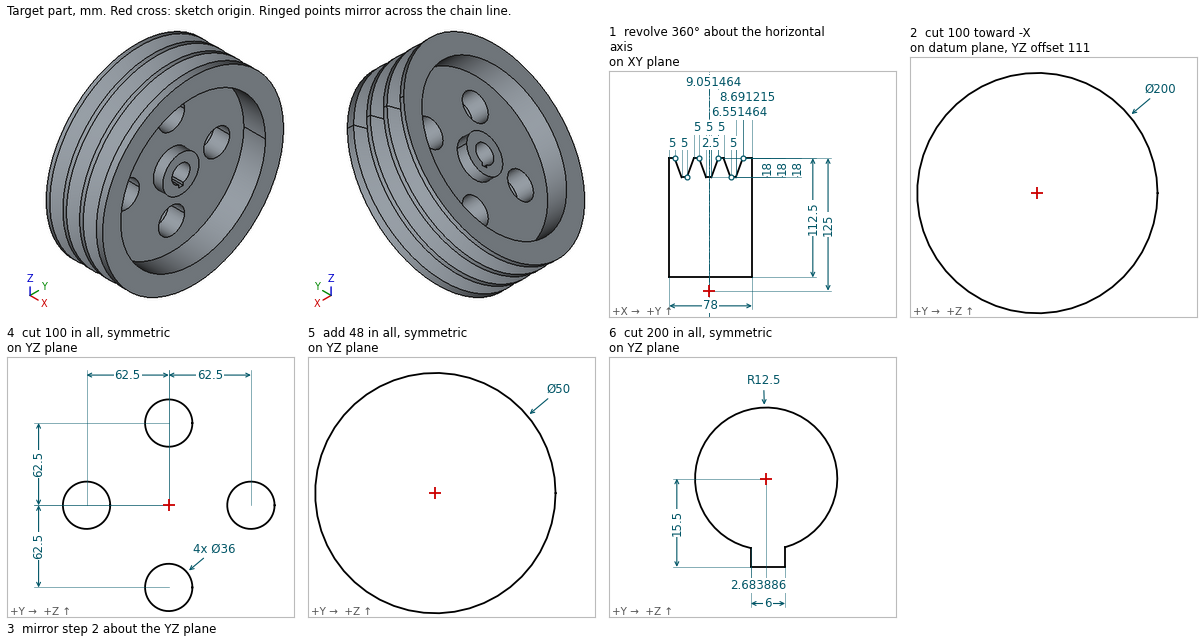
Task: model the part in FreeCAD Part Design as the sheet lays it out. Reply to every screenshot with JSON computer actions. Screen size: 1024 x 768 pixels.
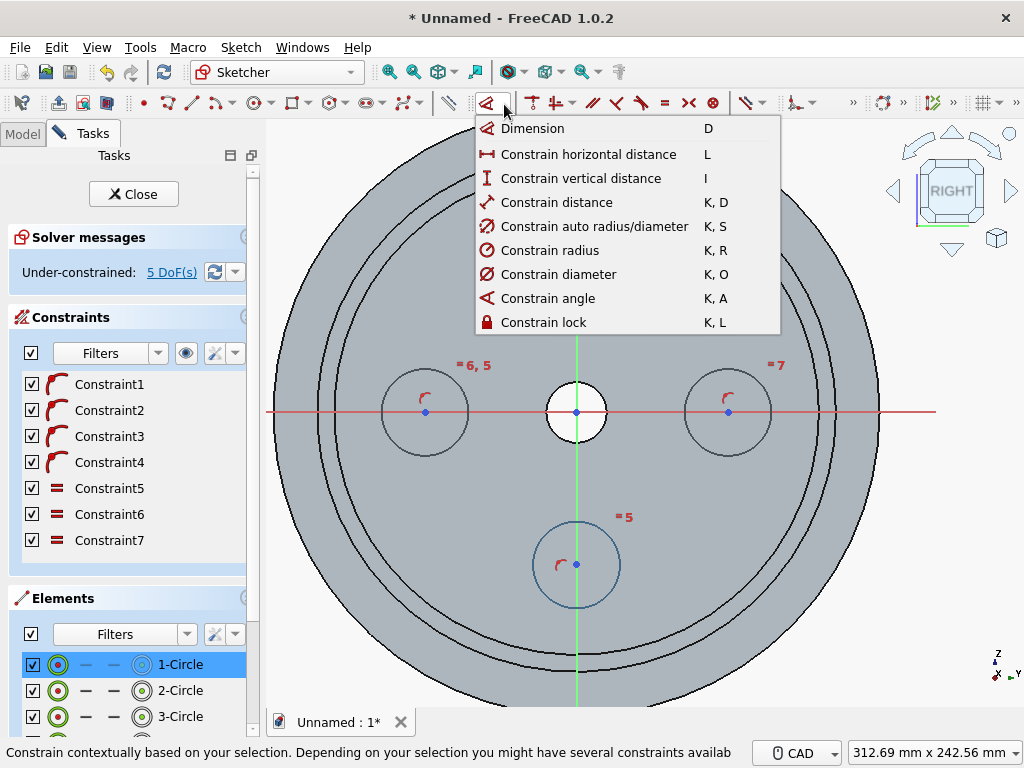
{"action": "left_click", "coordinate": [628, 274]}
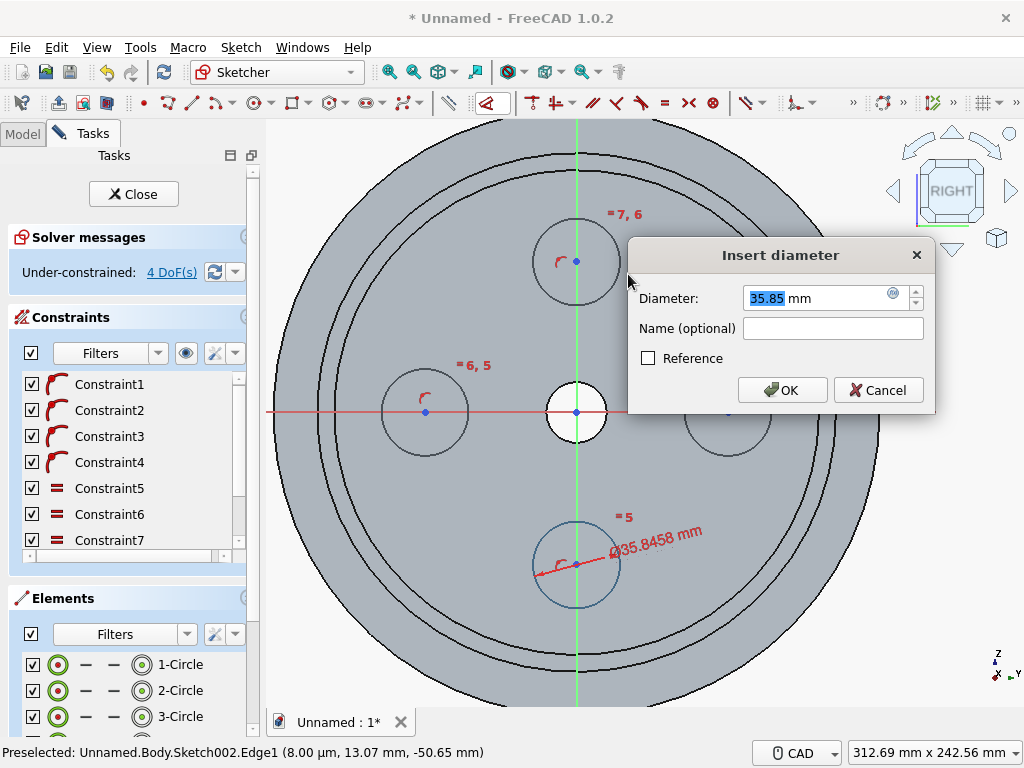
{"action": "type", "text": "36"}
{"action": "key", "text": "Return"}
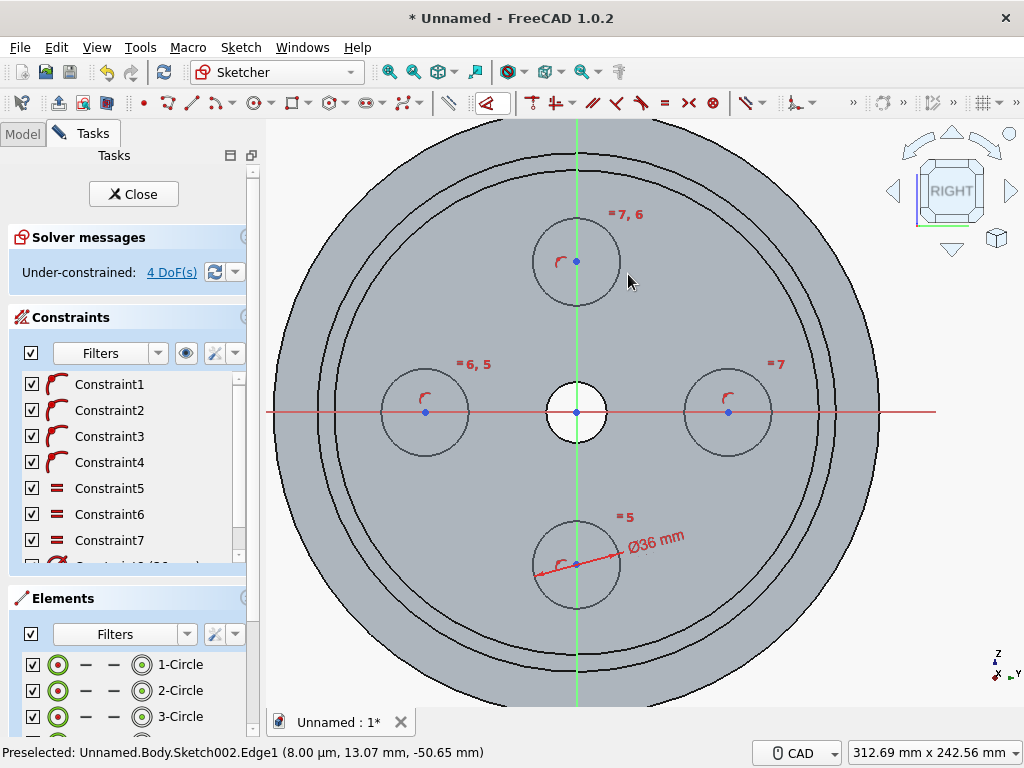
{"action": "left_click", "coordinate": [577, 565]}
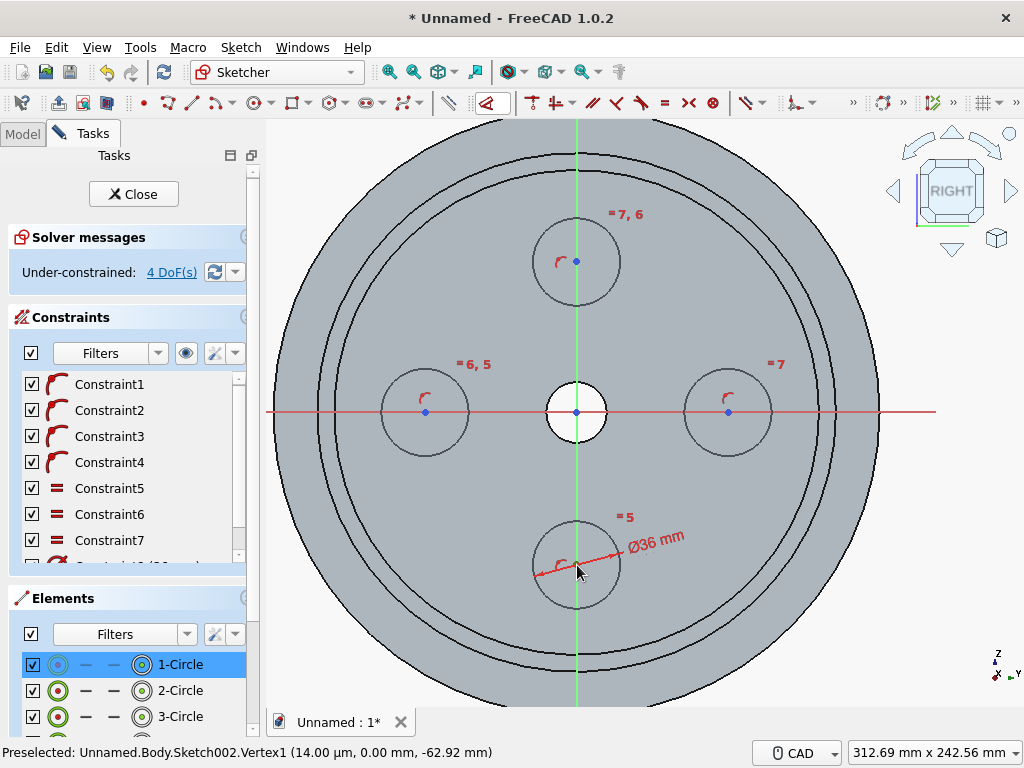
{"action": "key", "text": "i"}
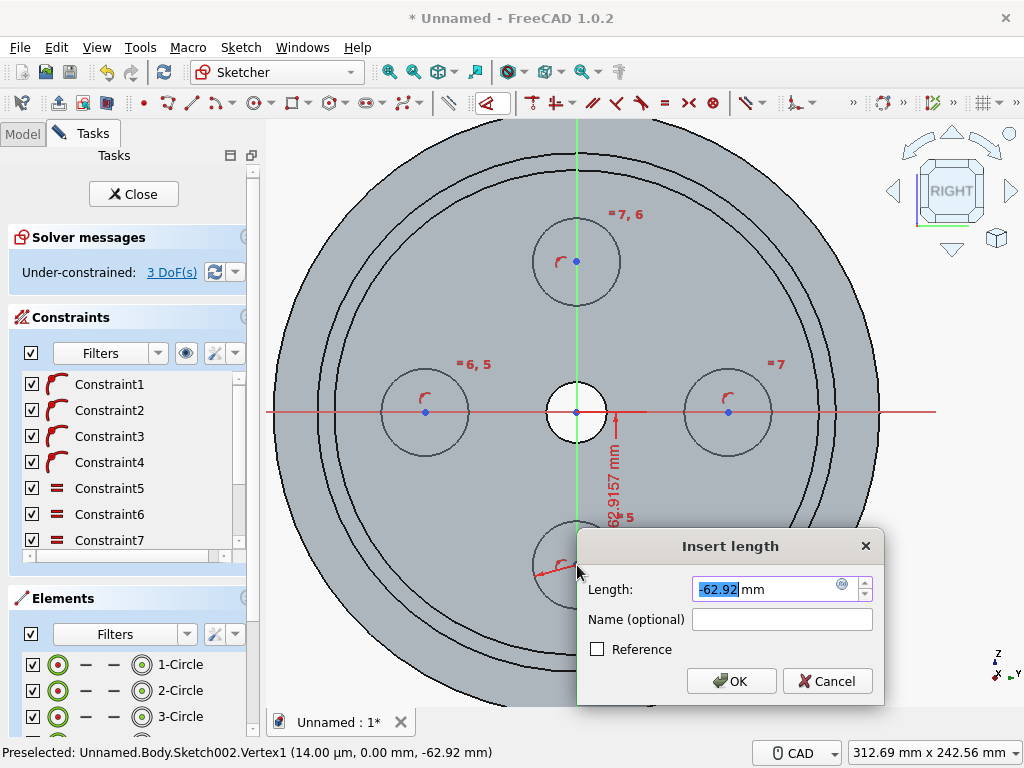
{"action": "type", "text": "-62.5"}
{"action": "key", "text": "Return"}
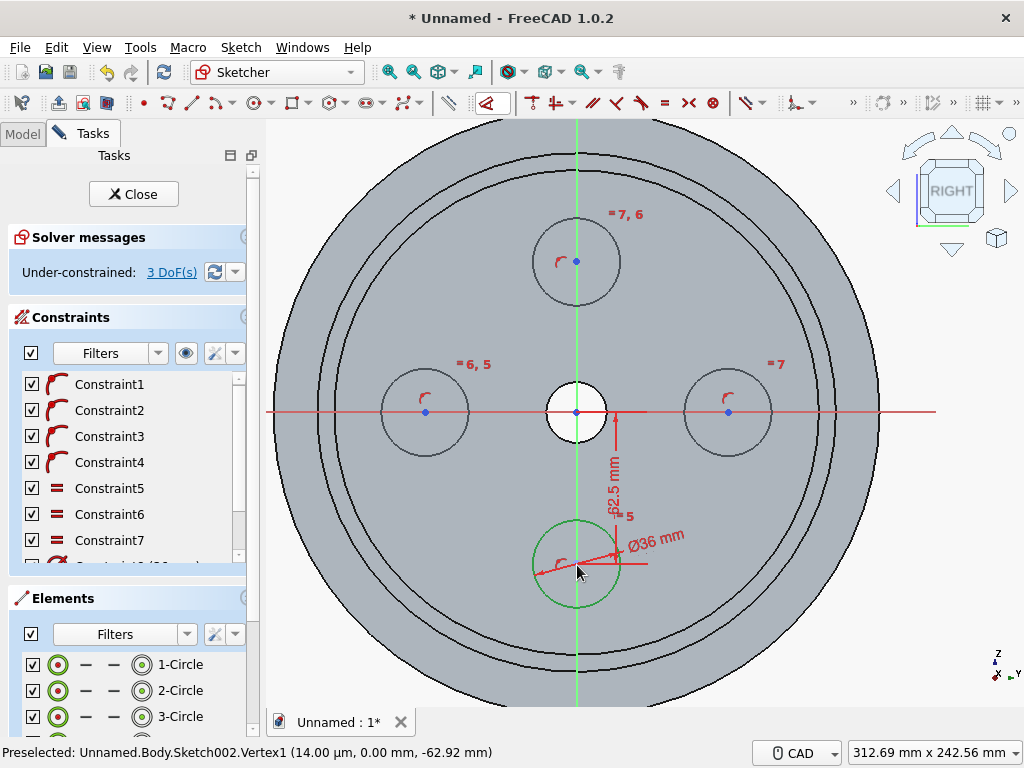
{"action": "left_click", "coordinate": [425, 412]}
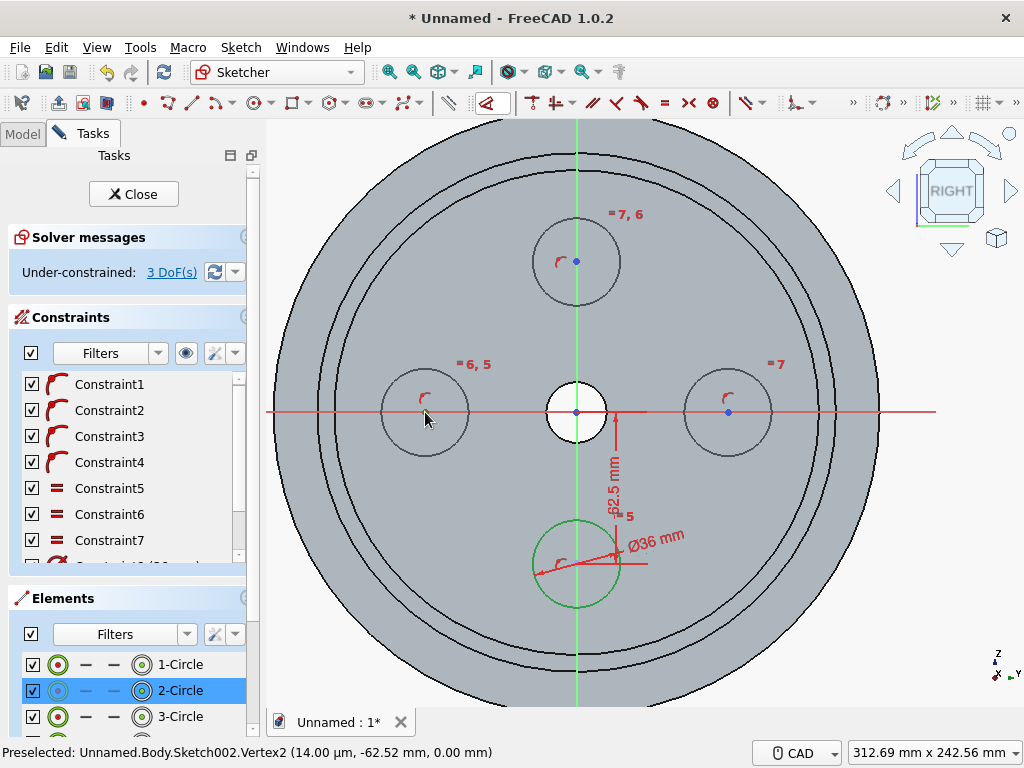
{"action": "left_click", "coordinate": [504, 104]}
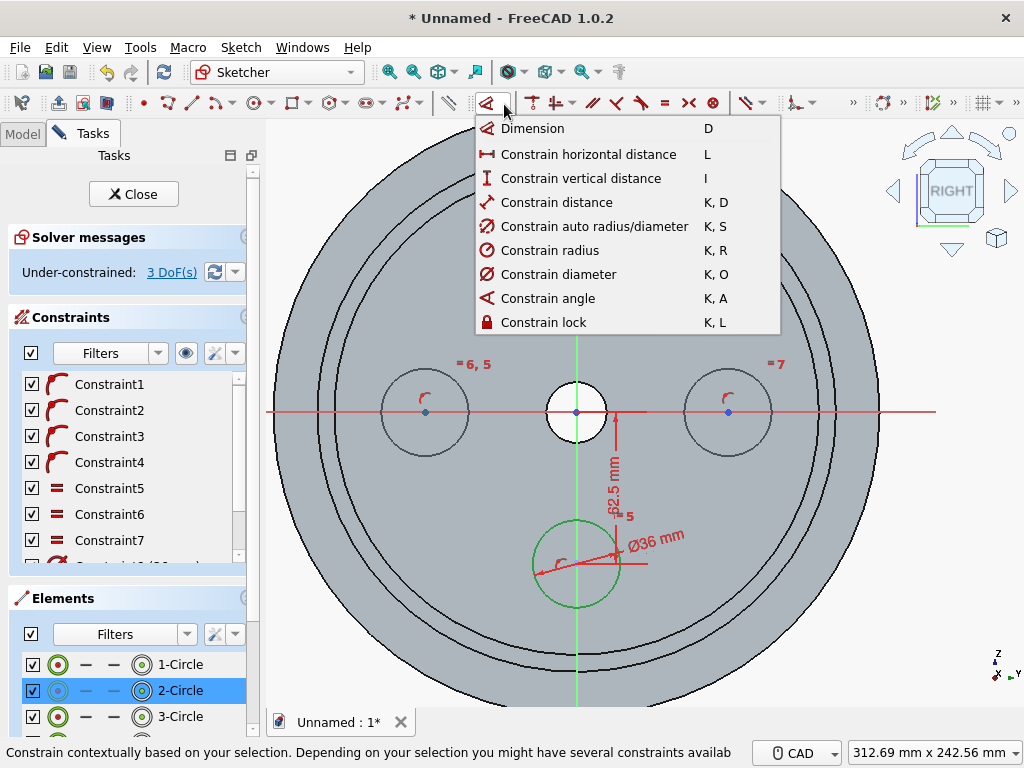
{"action": "left_click", "coordinate": [628, 154]}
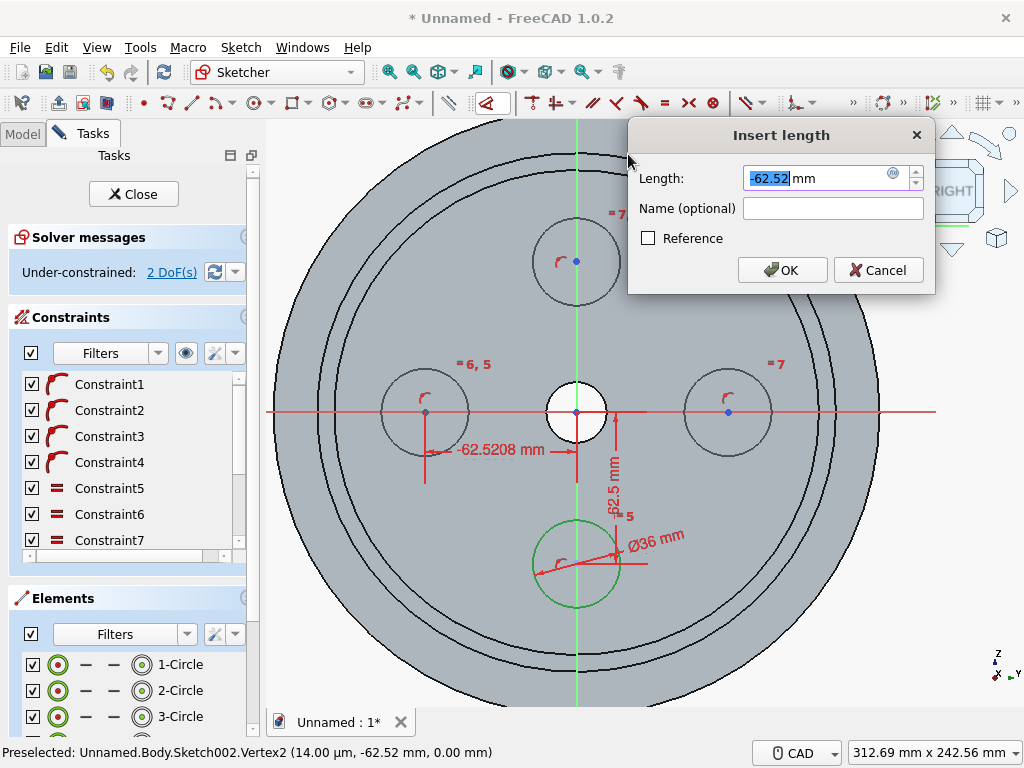
{"action": "type", "text": "-62.5"}
{"action": "key", "text": "Return"}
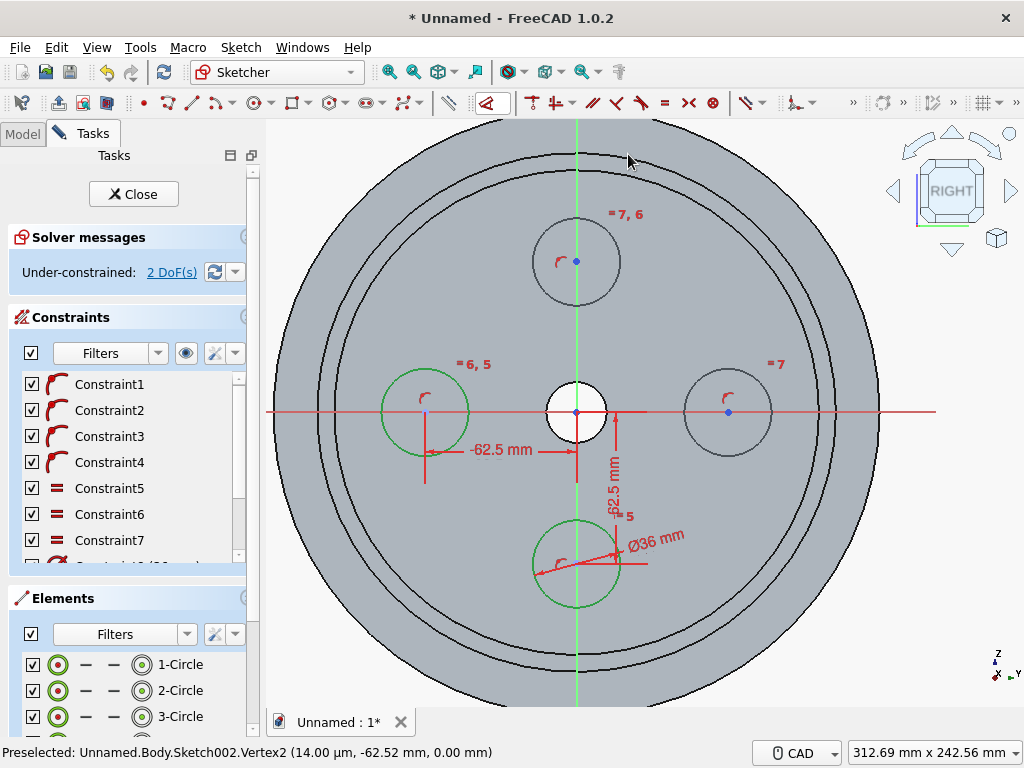
{"action": "left_click", "coordinate": [577, 262]}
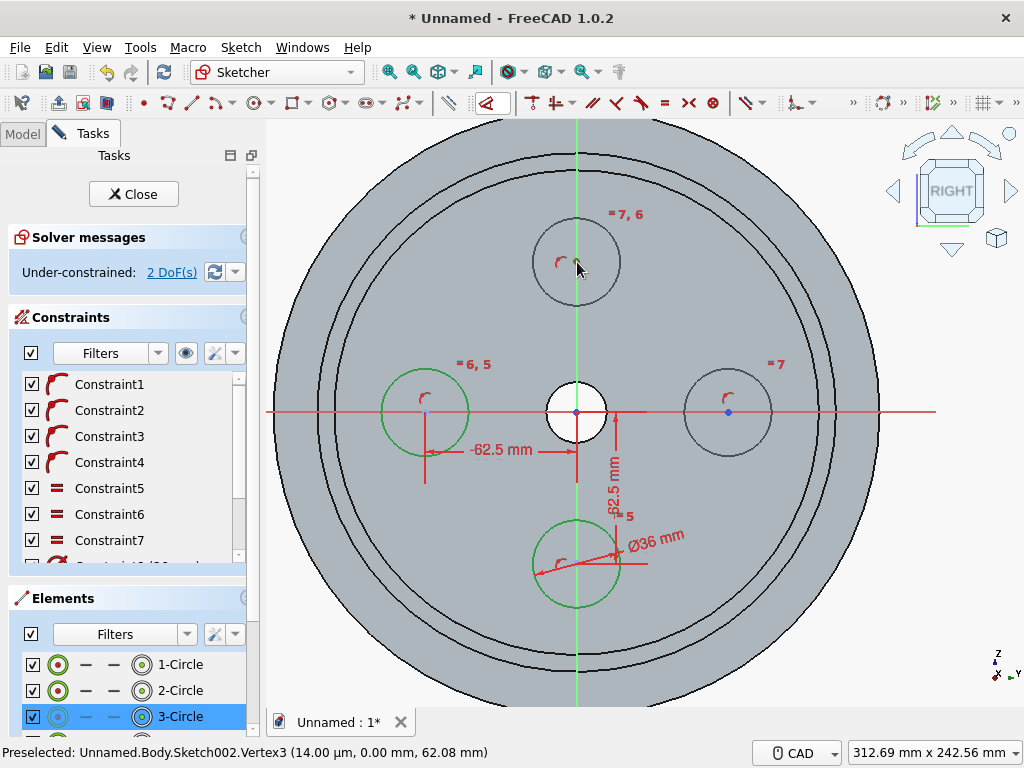
{"action": "key", "text": "i"}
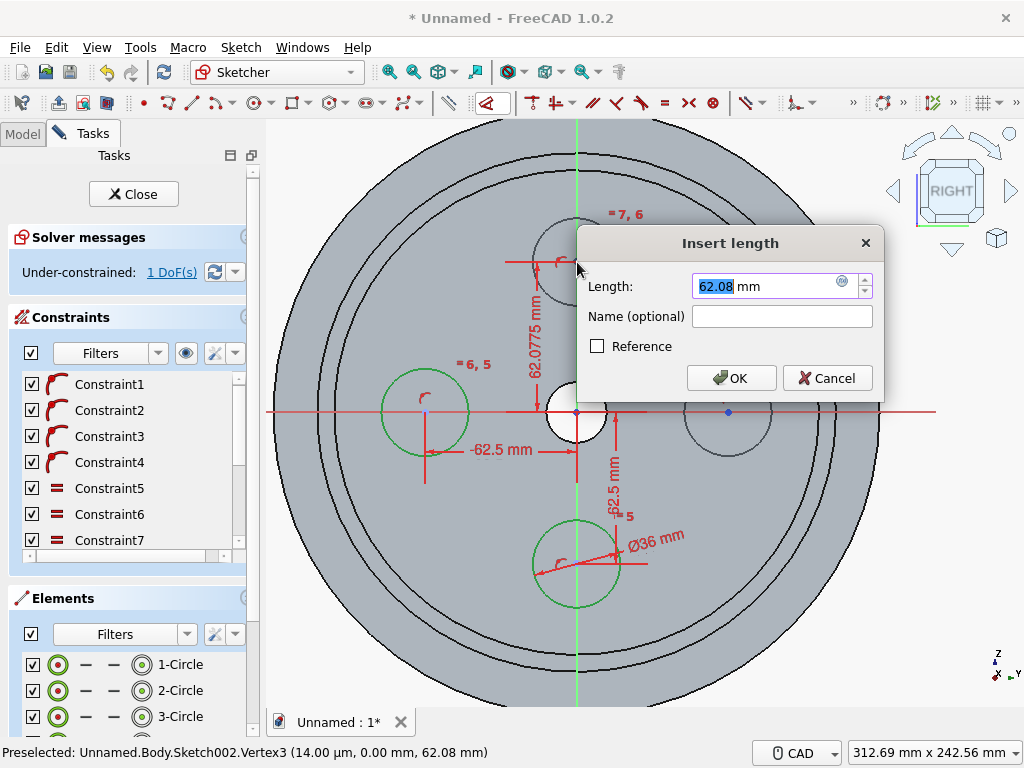
{"action": "type", "text": "62.5"}
{"action": "key", "text": "Return"}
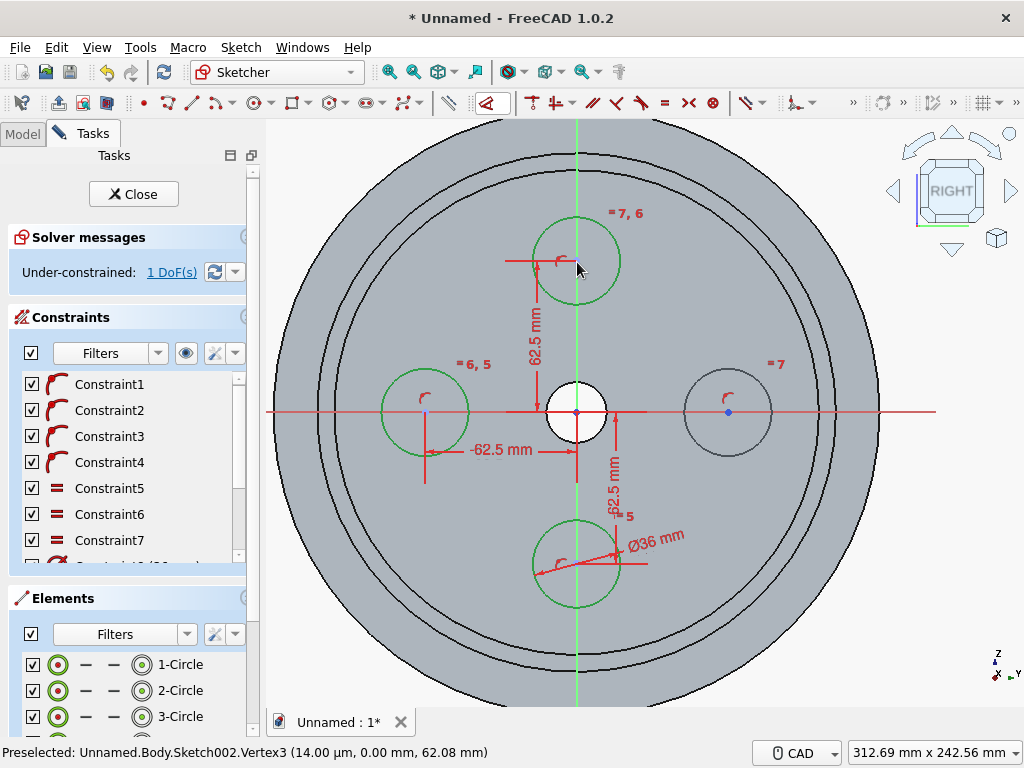
{"action": "left_click", "coordinate": [728, 412]}